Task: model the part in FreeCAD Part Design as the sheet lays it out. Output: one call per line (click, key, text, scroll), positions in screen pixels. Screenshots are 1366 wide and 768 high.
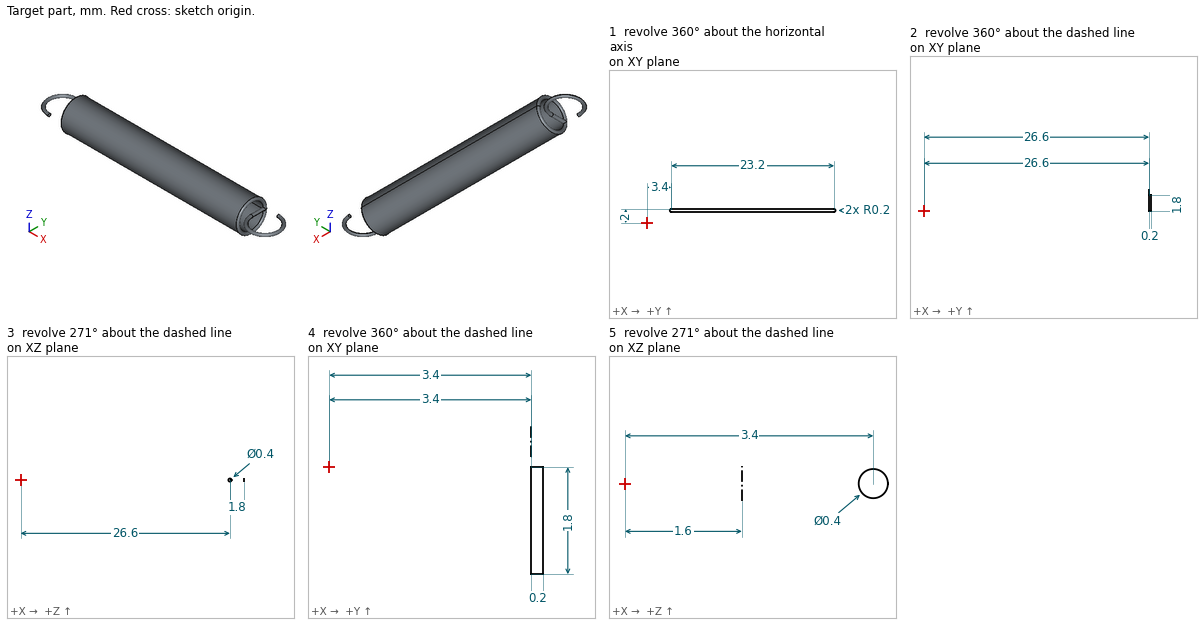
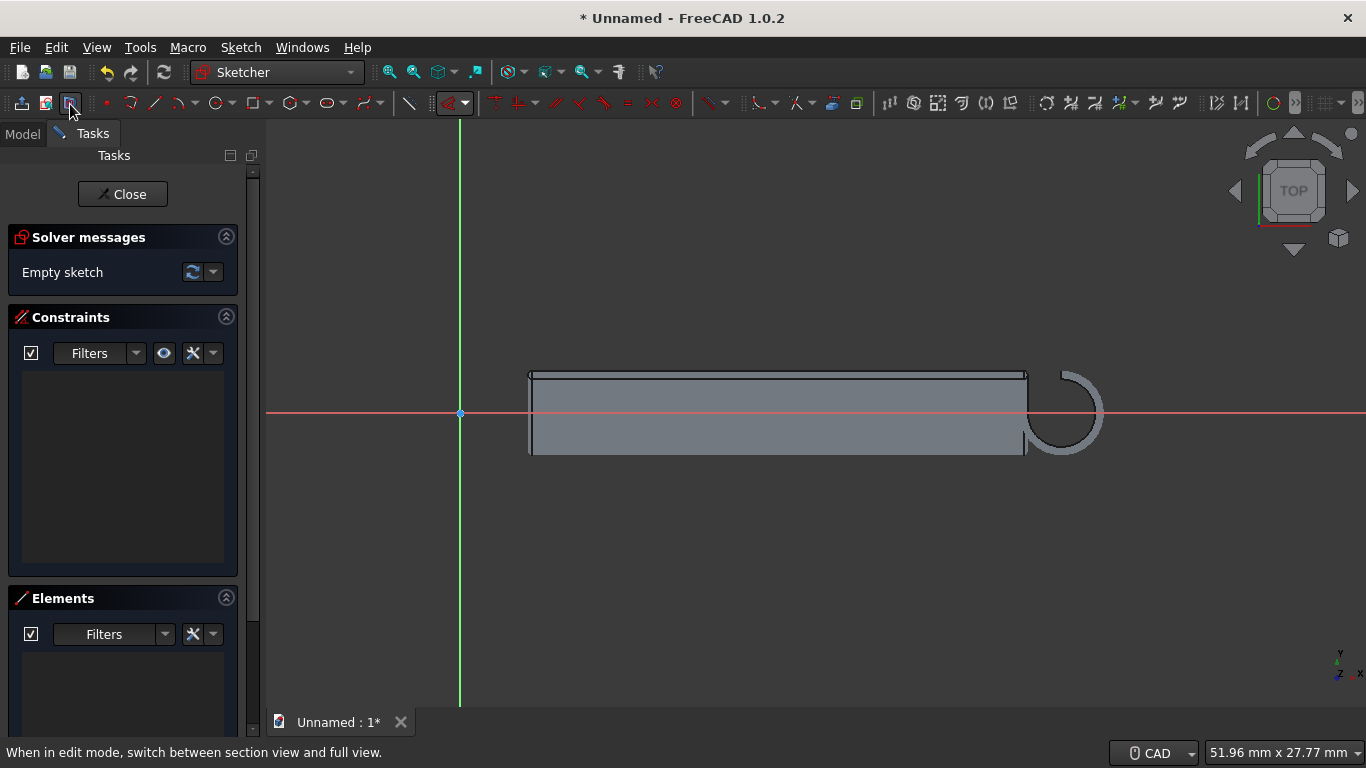
scroll(459, 426, up, 10)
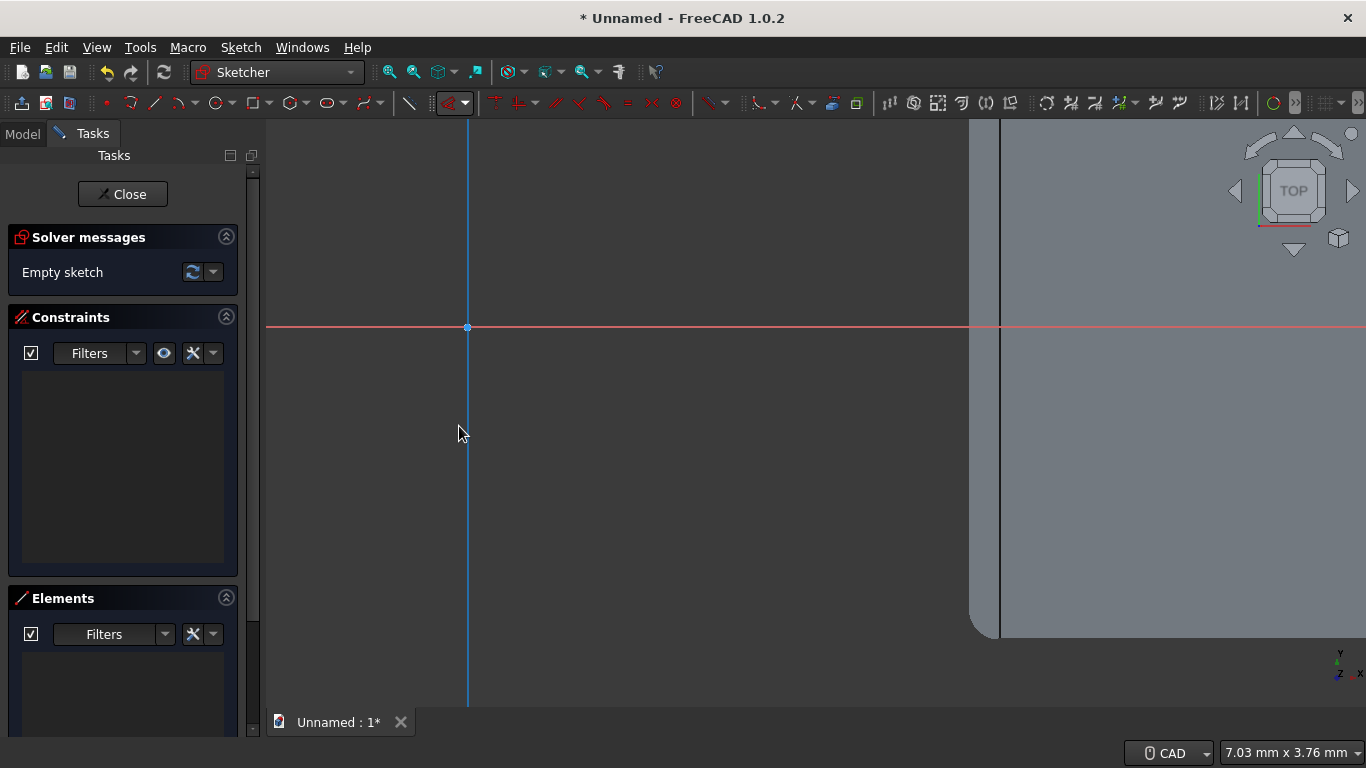
click(254, 104)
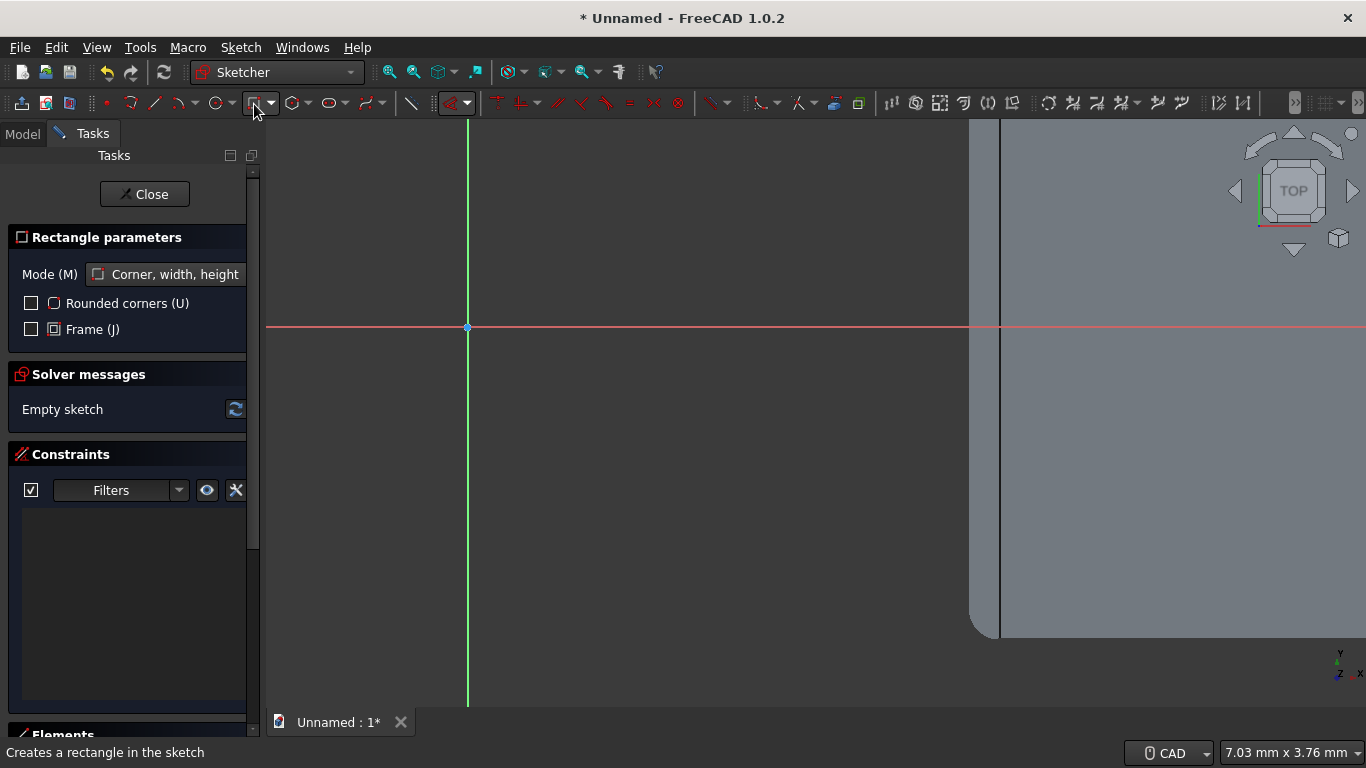
click(1000, 327)
click(1031, 609)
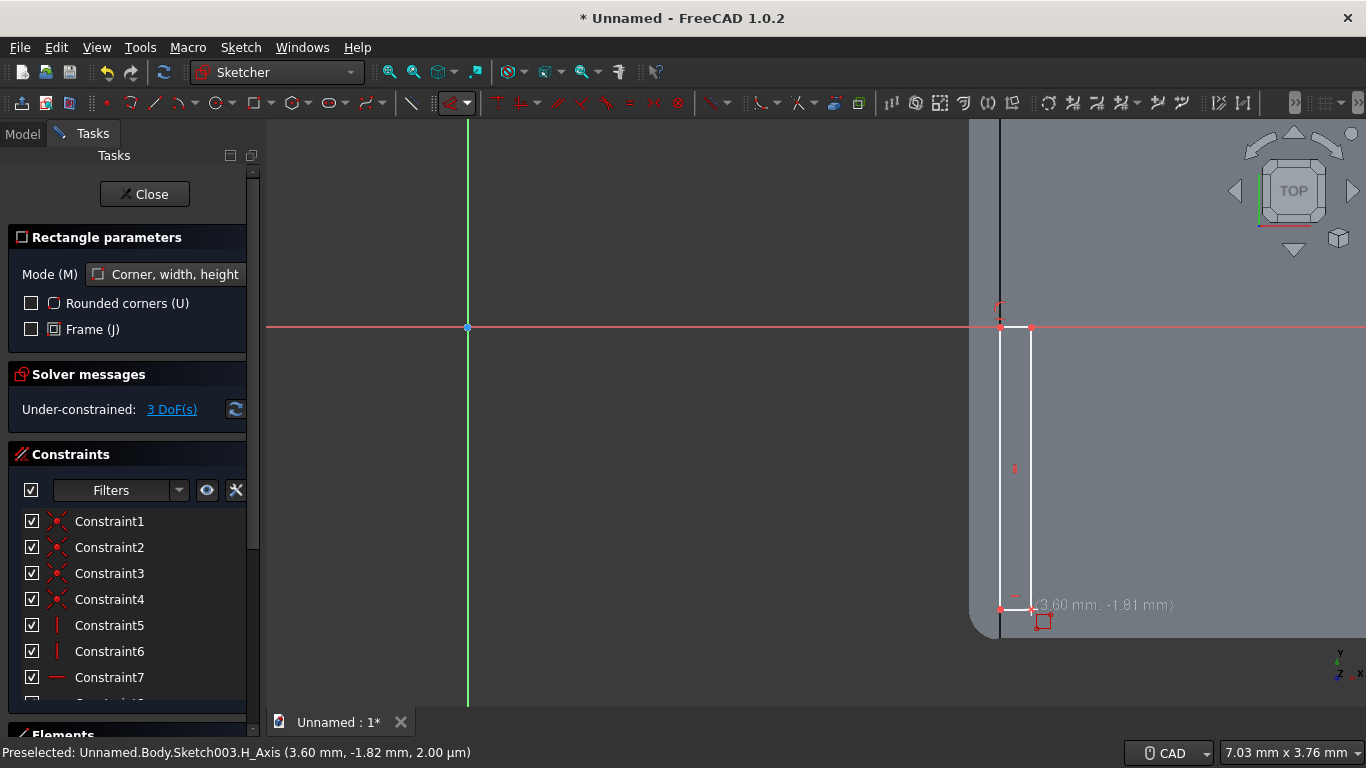
click(156, 104)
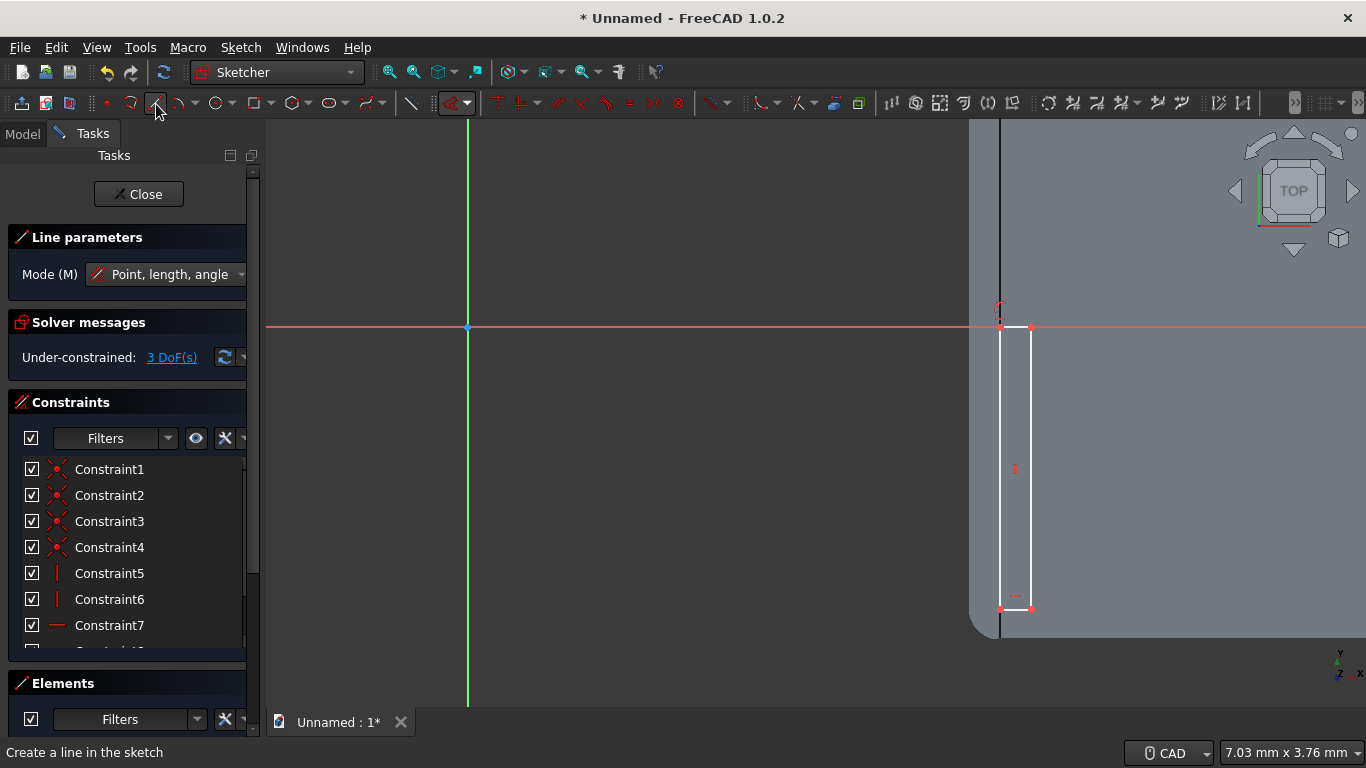
click(1000, 299)
click(1000, 214)
key(Escape)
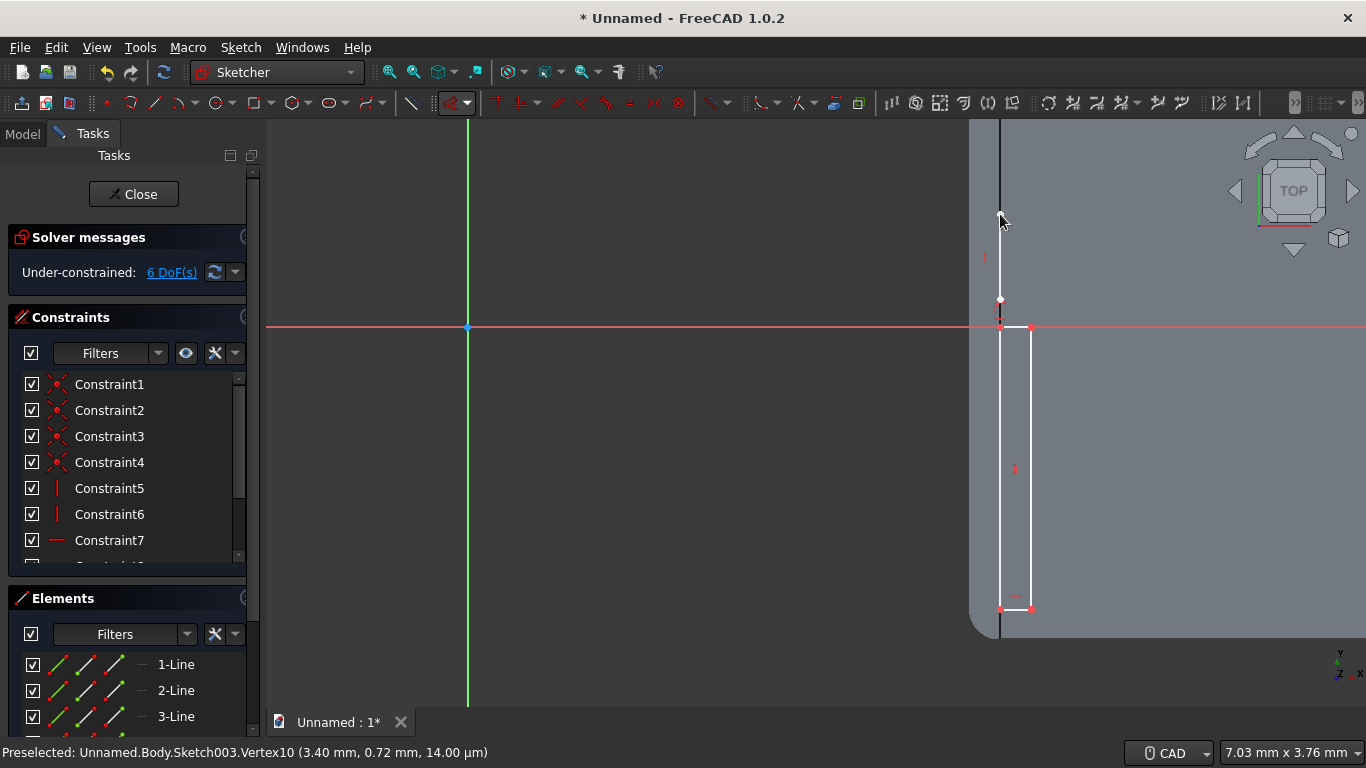
click(1000, 274)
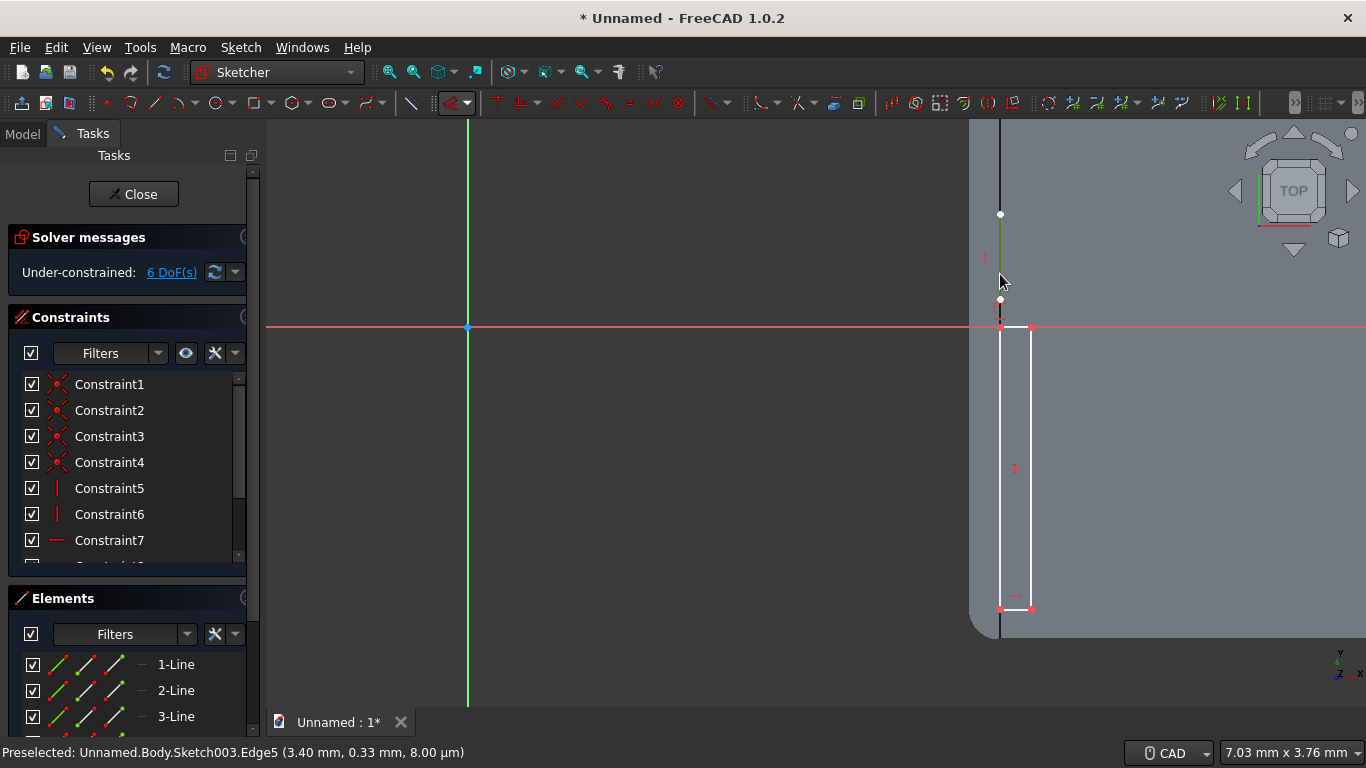
click(412, 104)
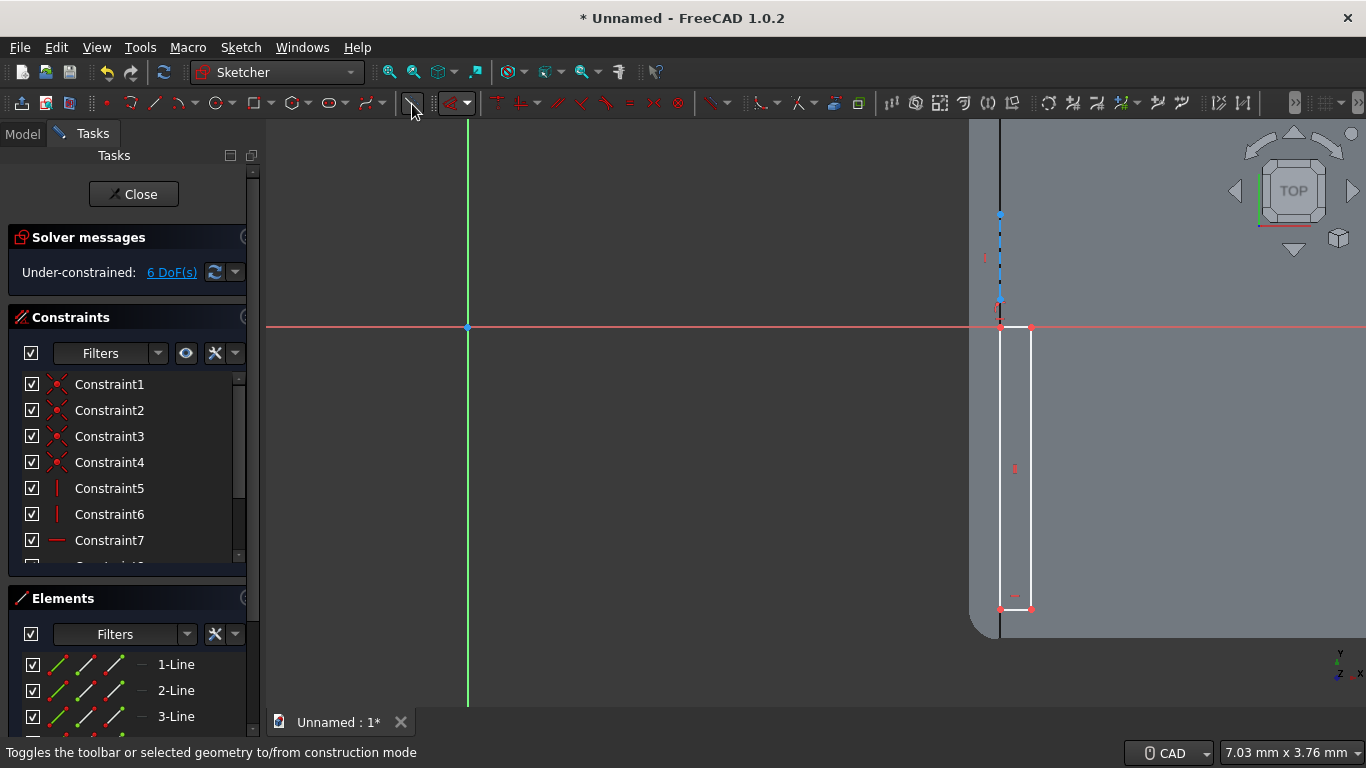
click(1000, 412)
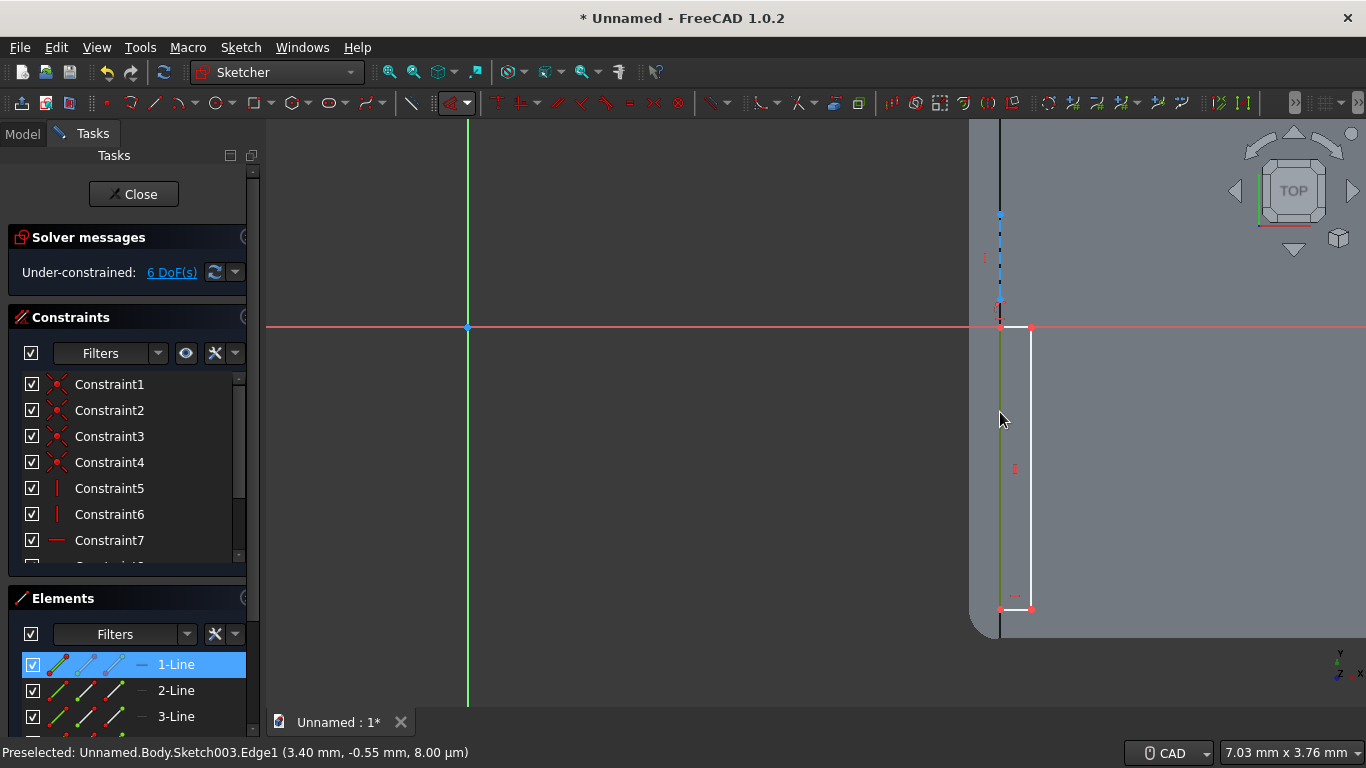
key(i)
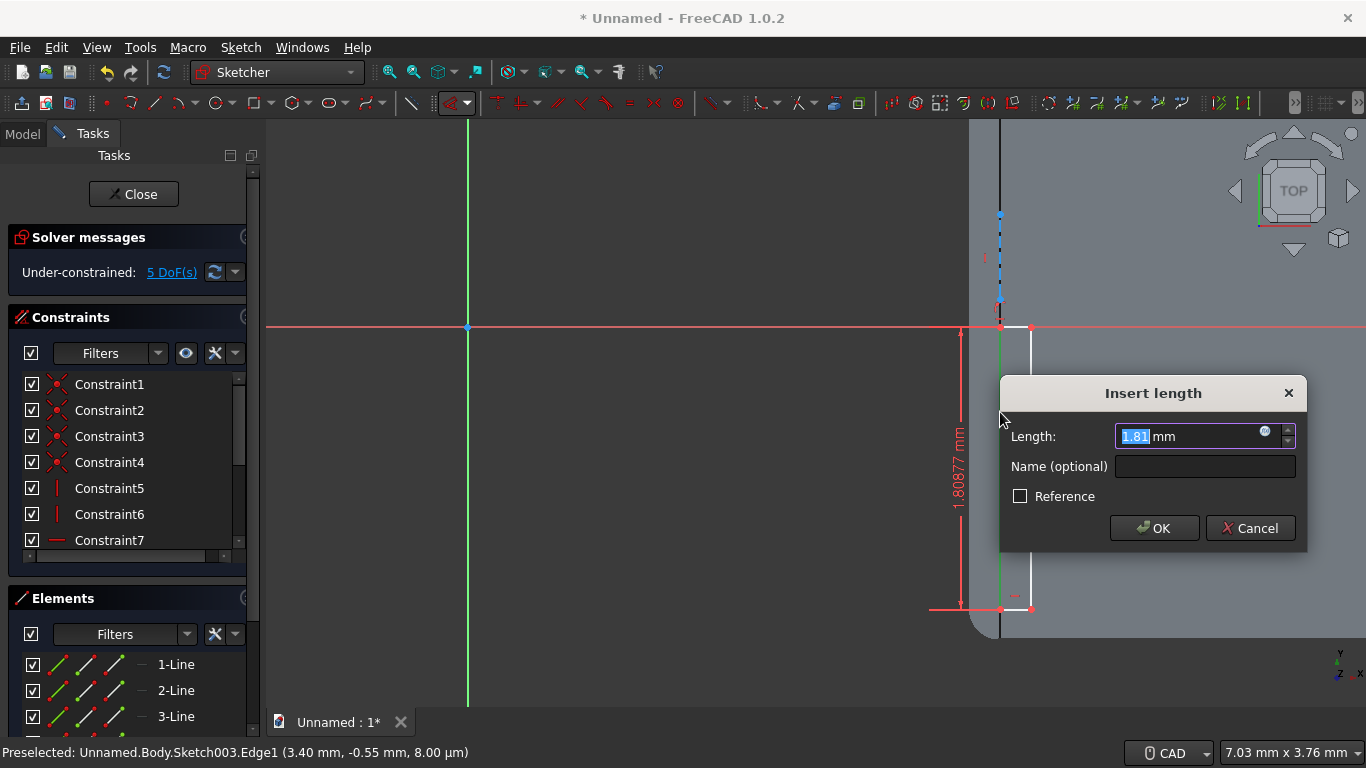
text(1.8)
key(Return)